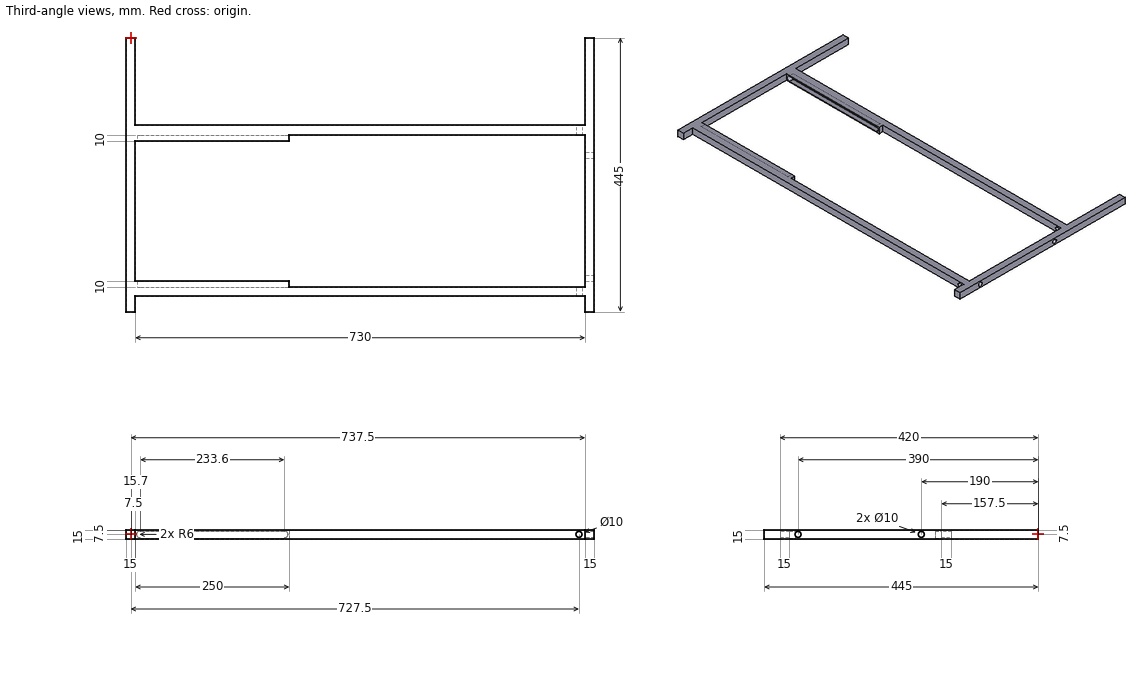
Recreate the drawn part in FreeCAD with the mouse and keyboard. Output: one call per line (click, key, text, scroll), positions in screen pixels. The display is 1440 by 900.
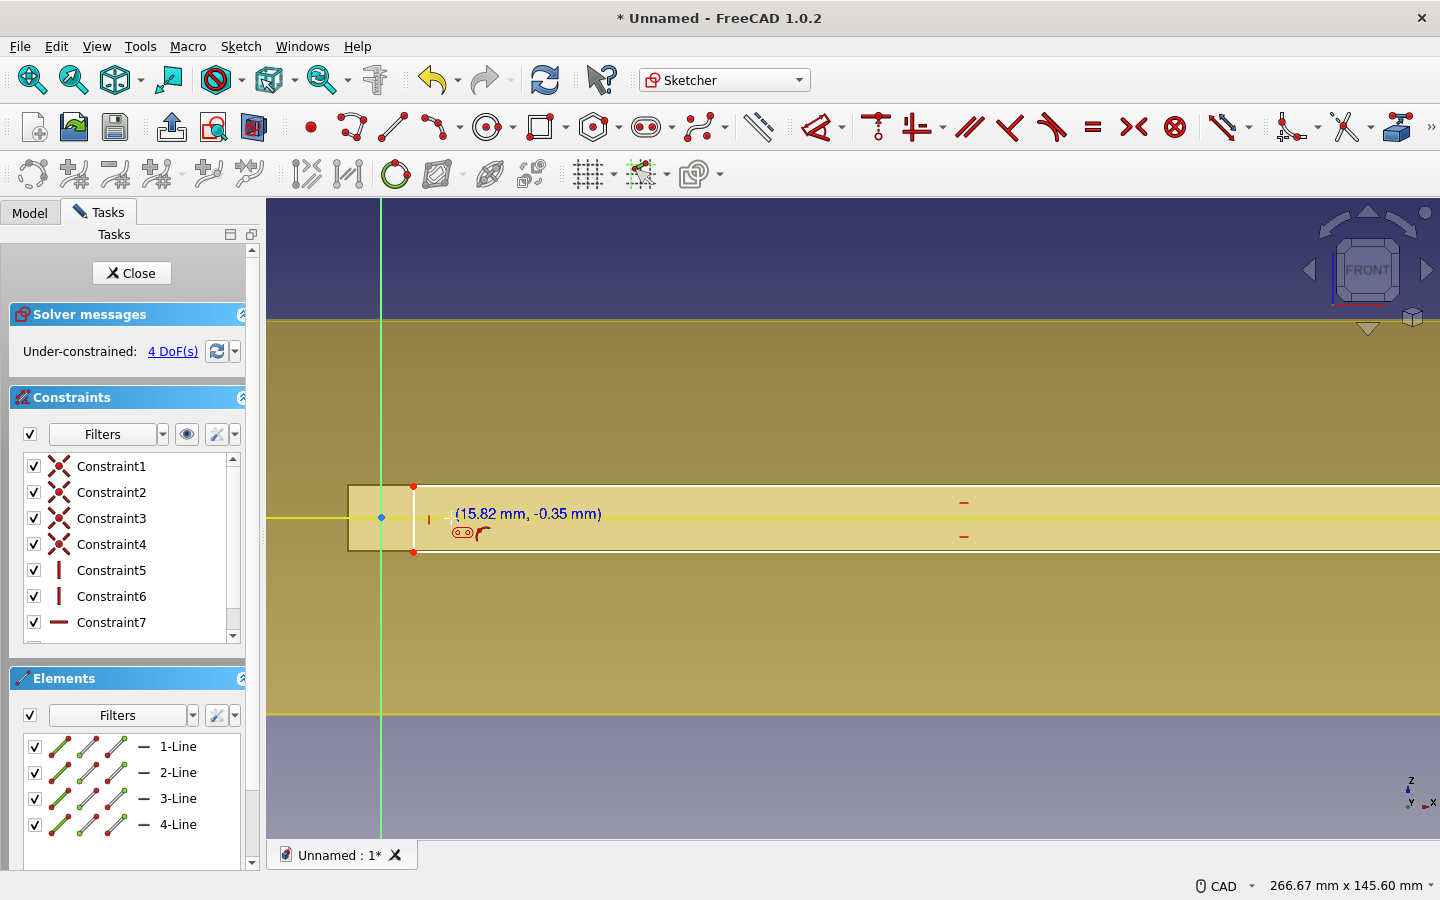
click(450, 518)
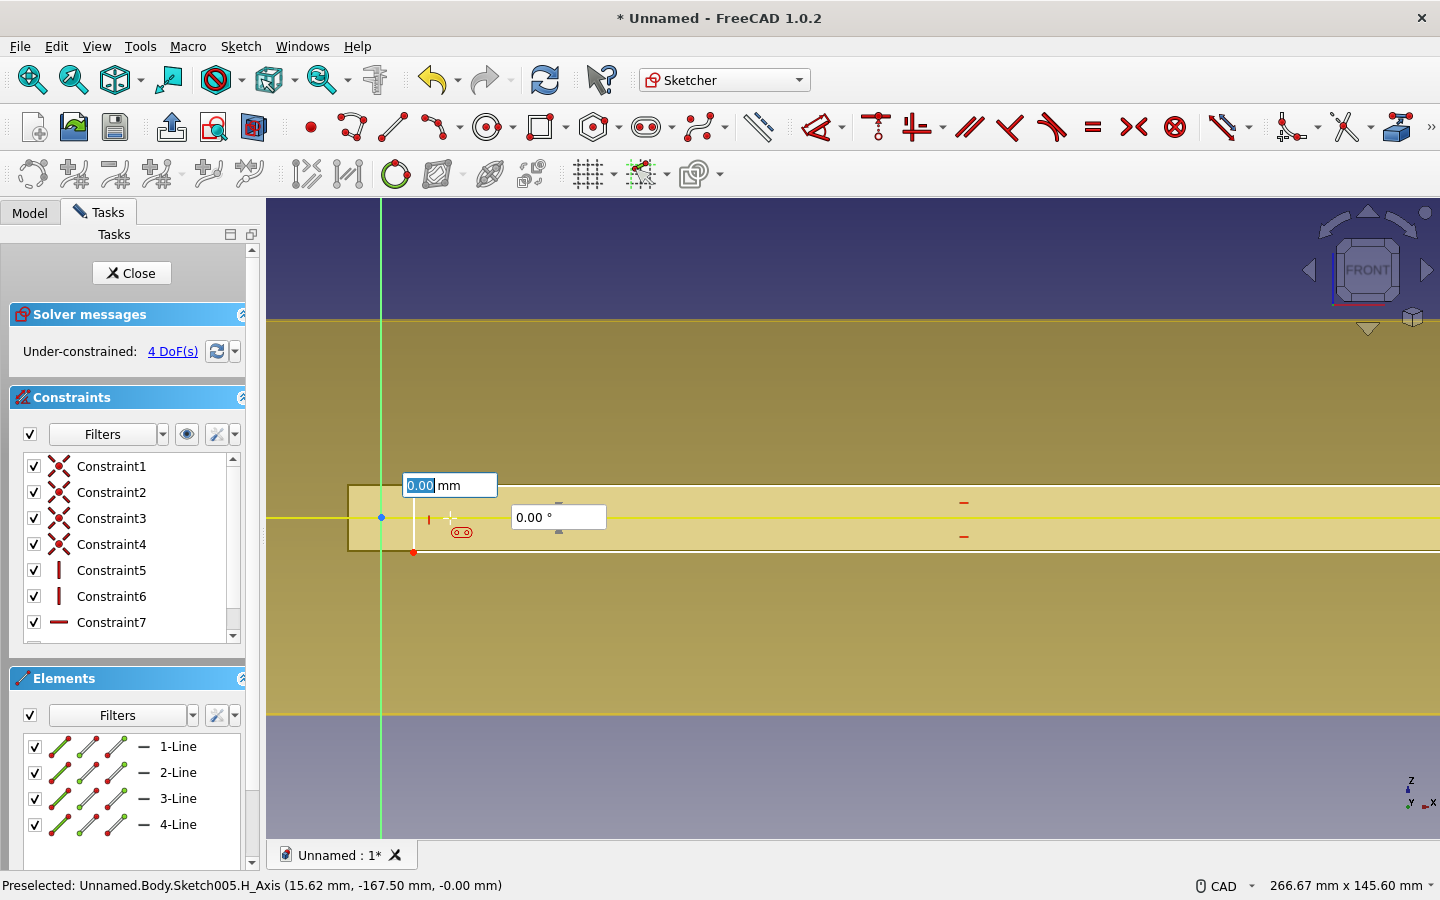
scroll(452, 520, down, 2)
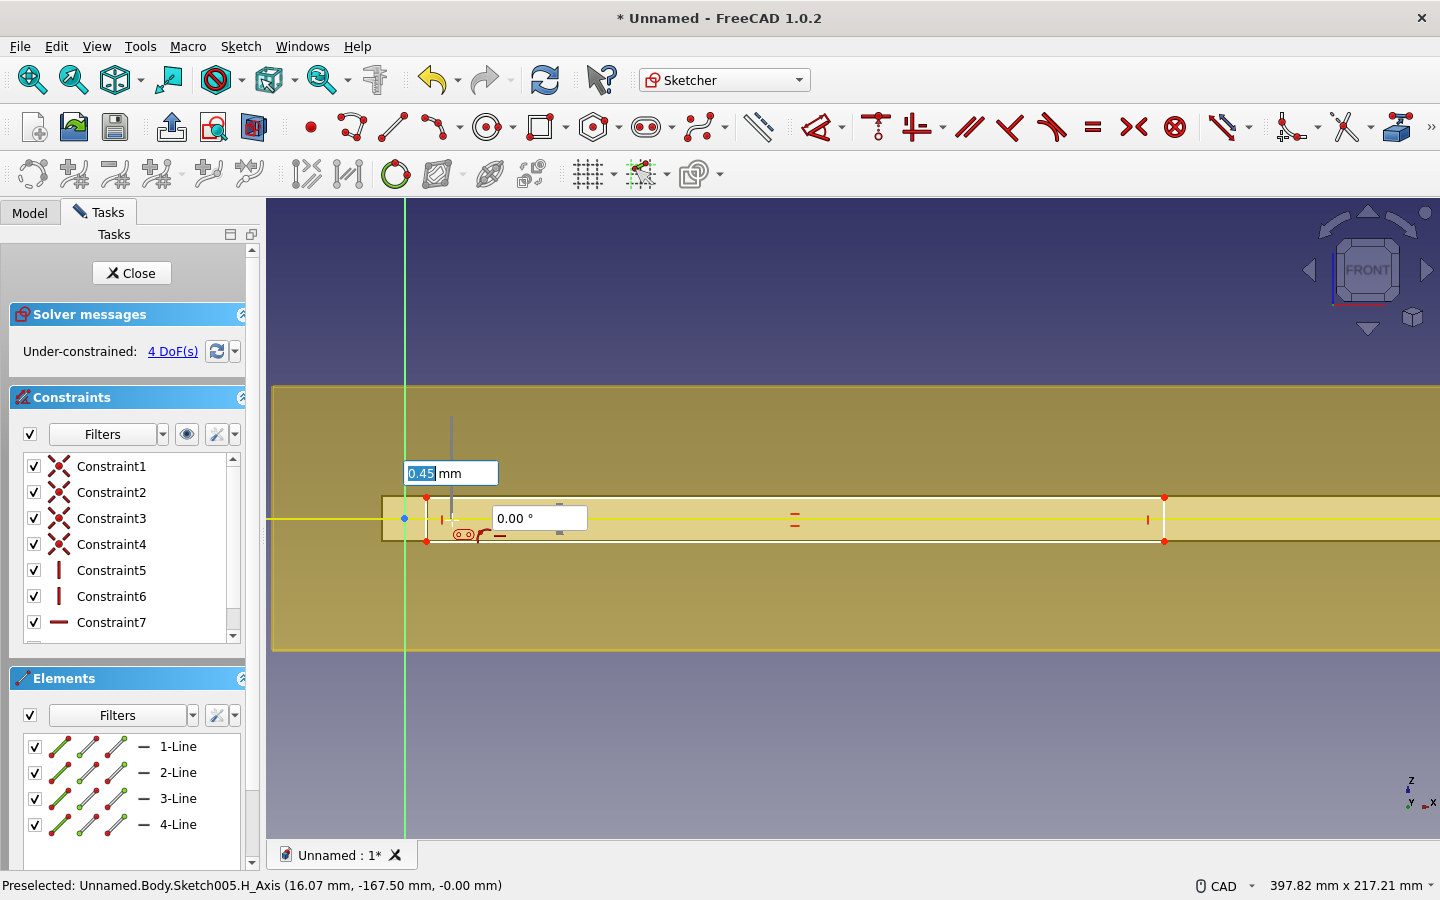
click(1140, 510)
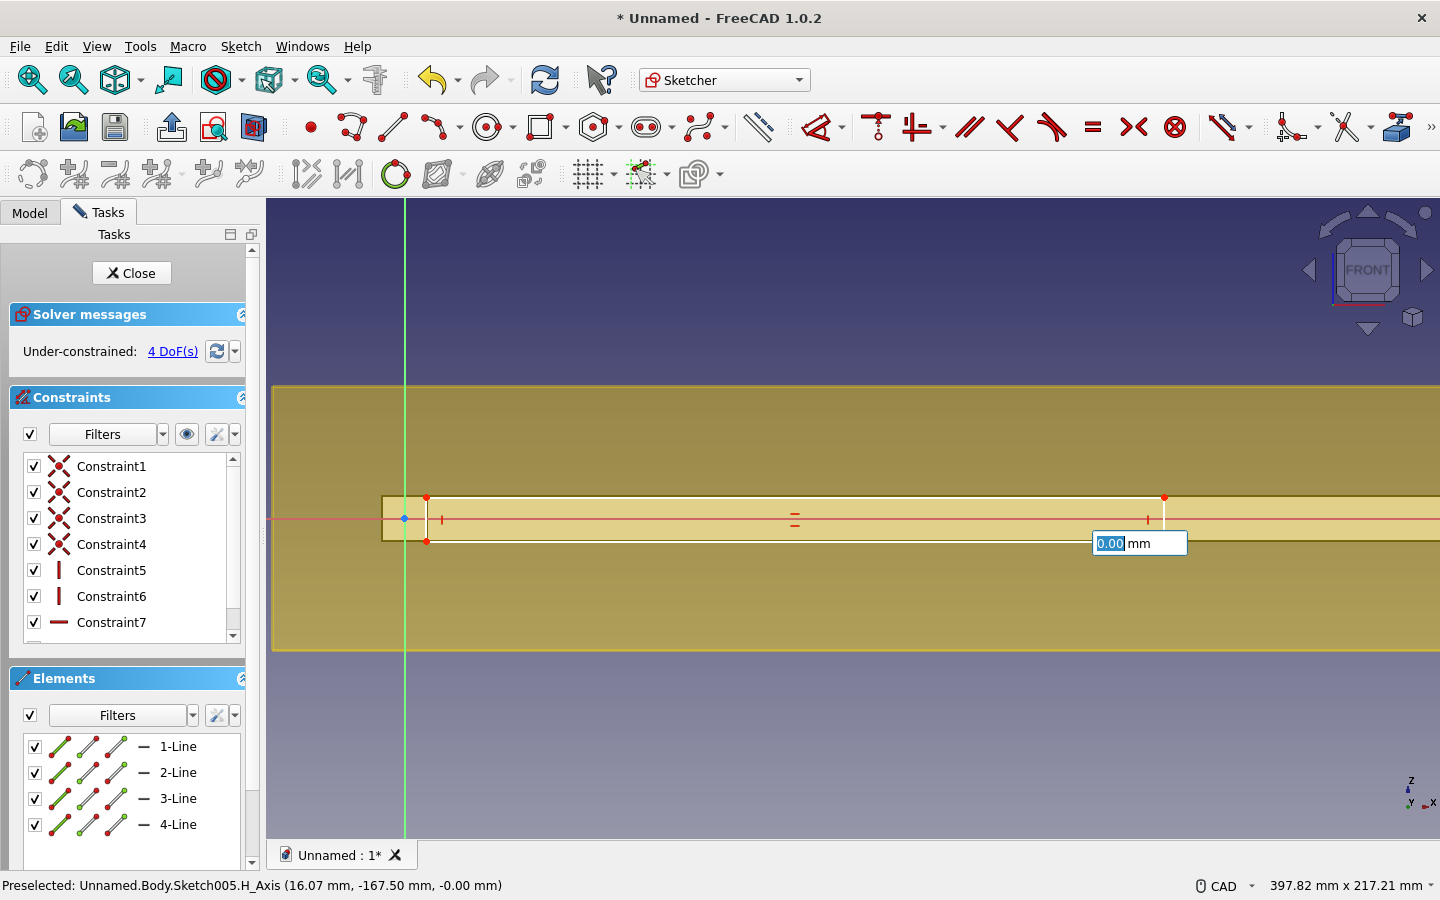
scroll(796, 536, up, 7)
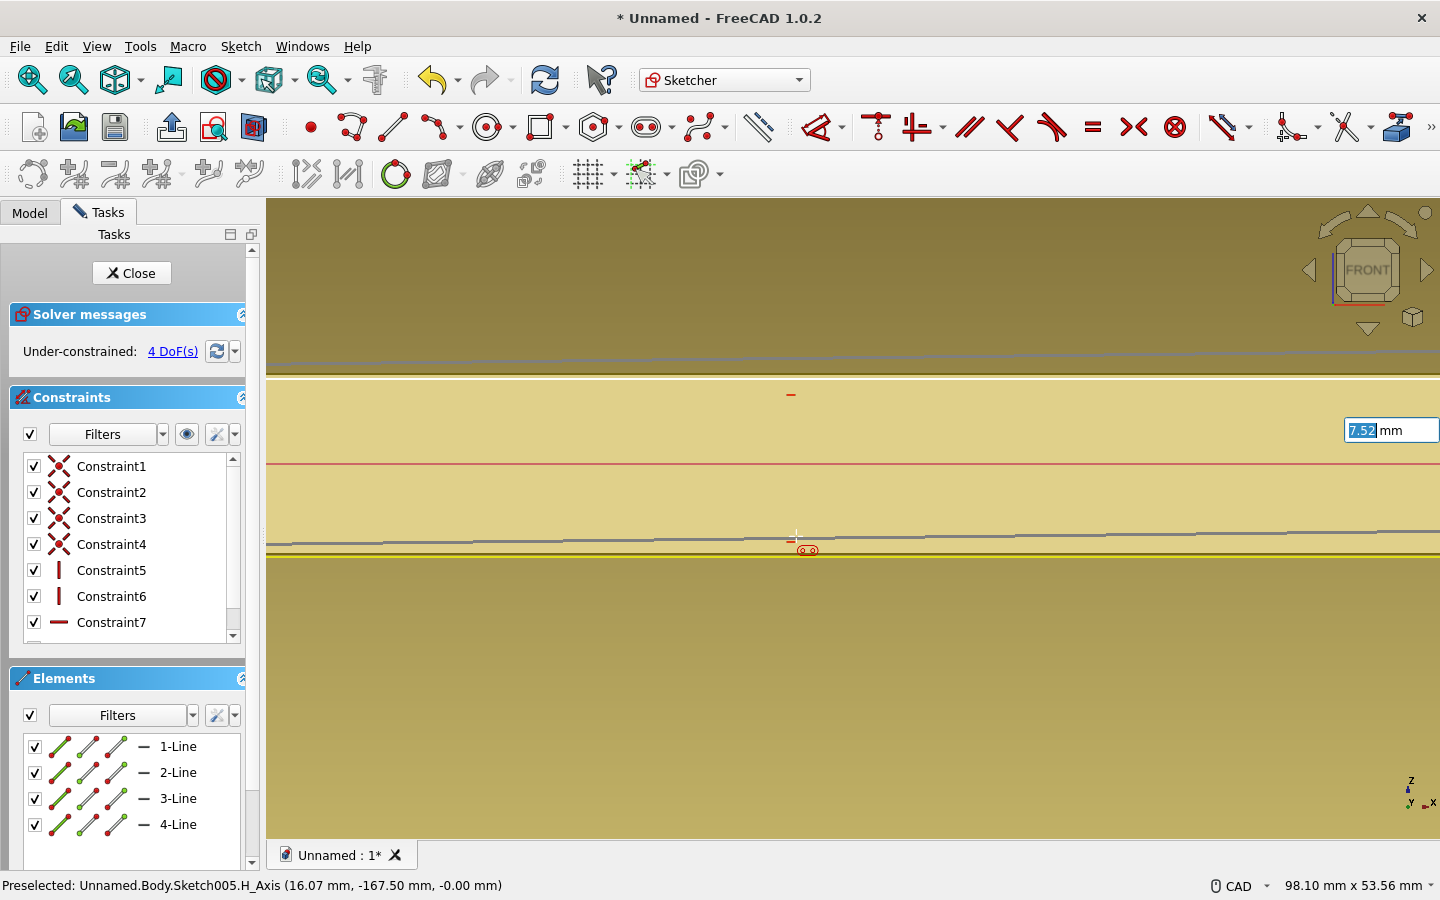
click(793, 536)
key(Escape)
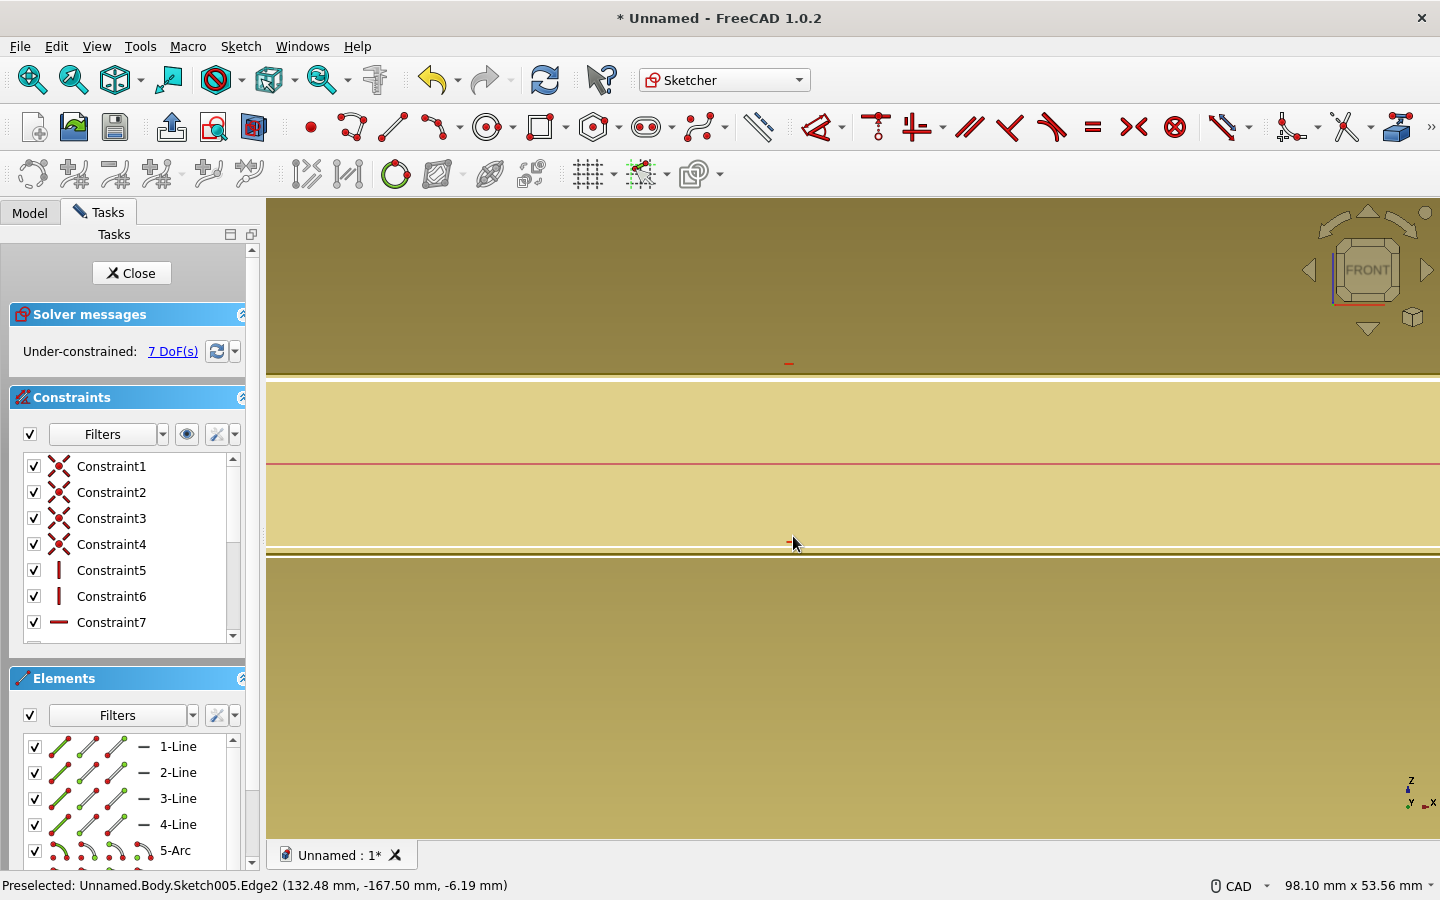
click(816, 128)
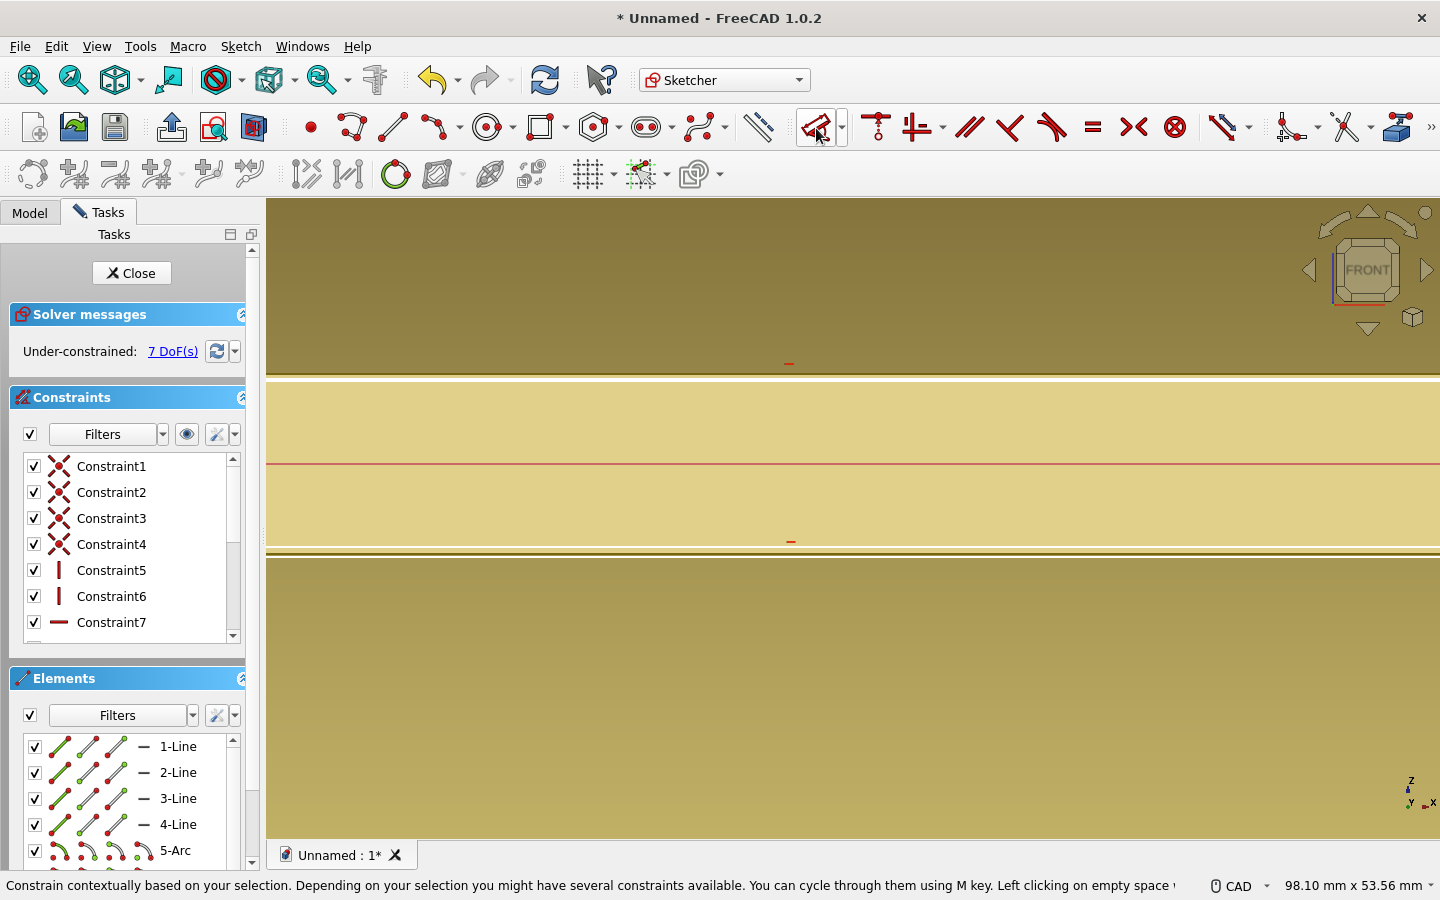
scroll(796, 536, down, 7)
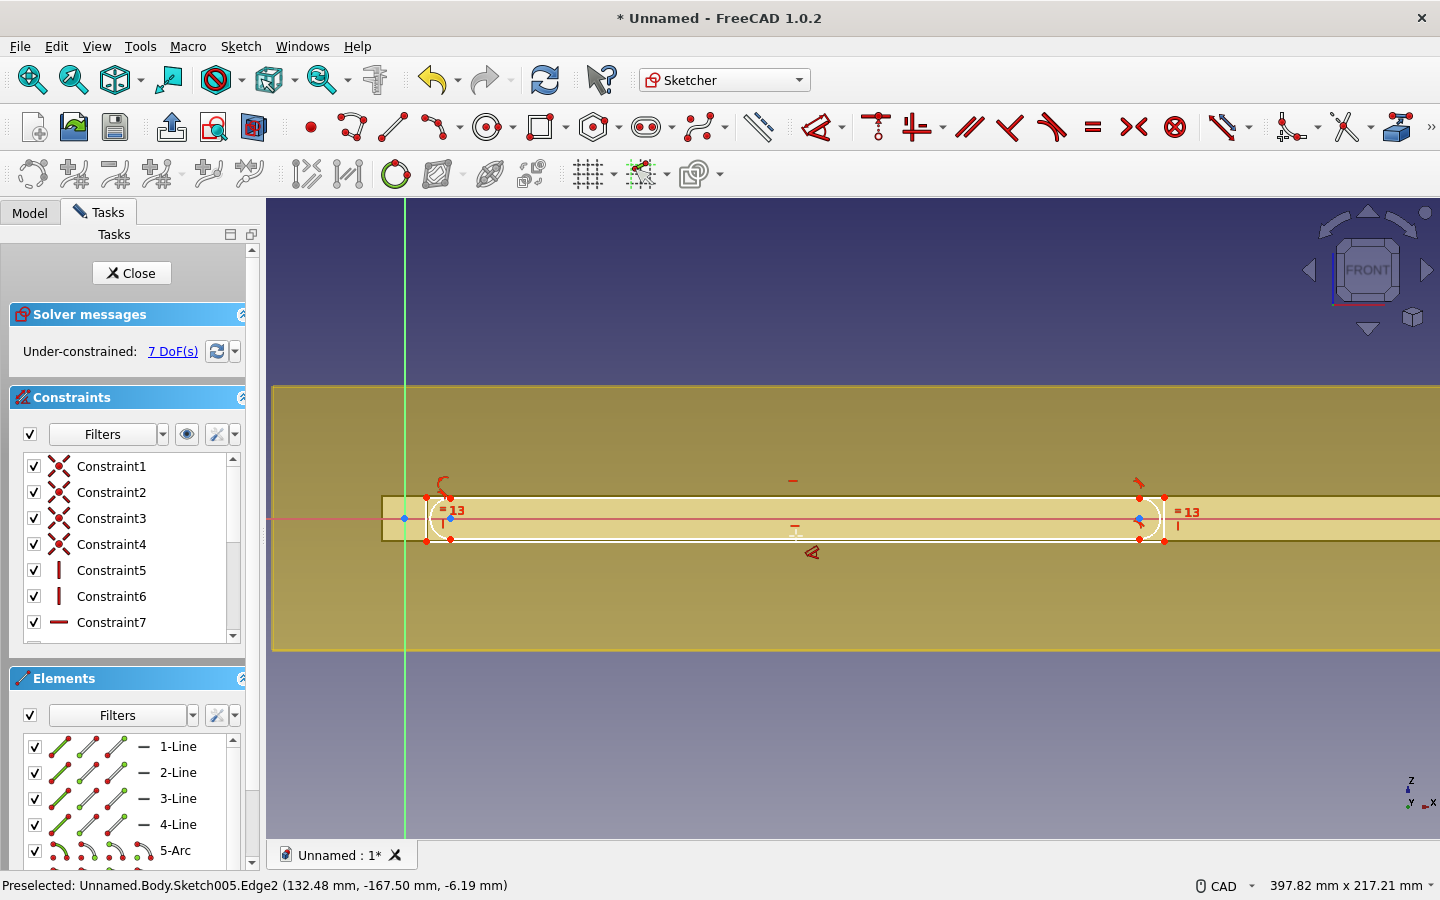
scroll(434, 507, up, 5)